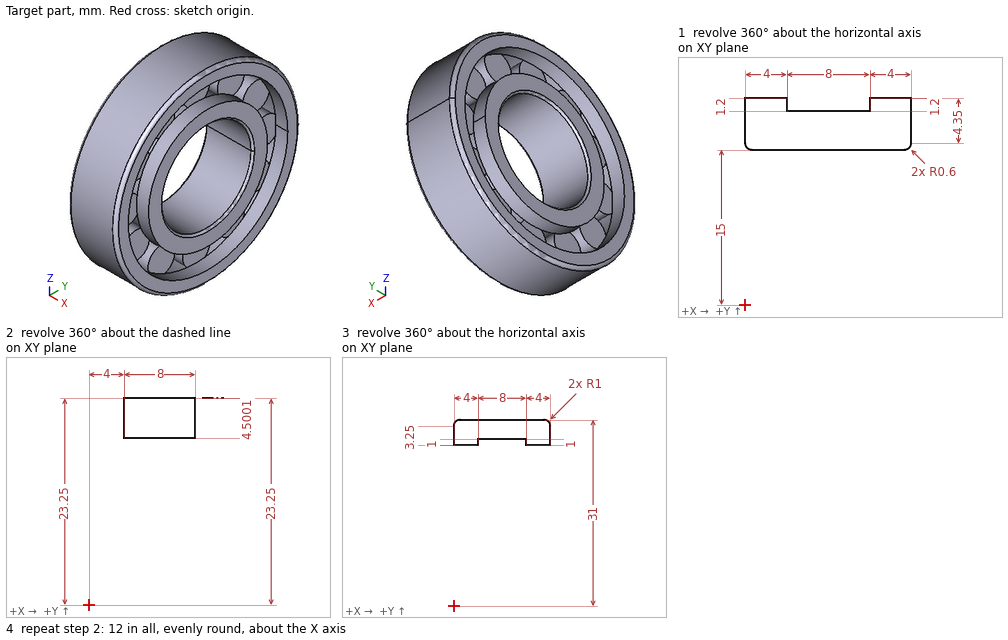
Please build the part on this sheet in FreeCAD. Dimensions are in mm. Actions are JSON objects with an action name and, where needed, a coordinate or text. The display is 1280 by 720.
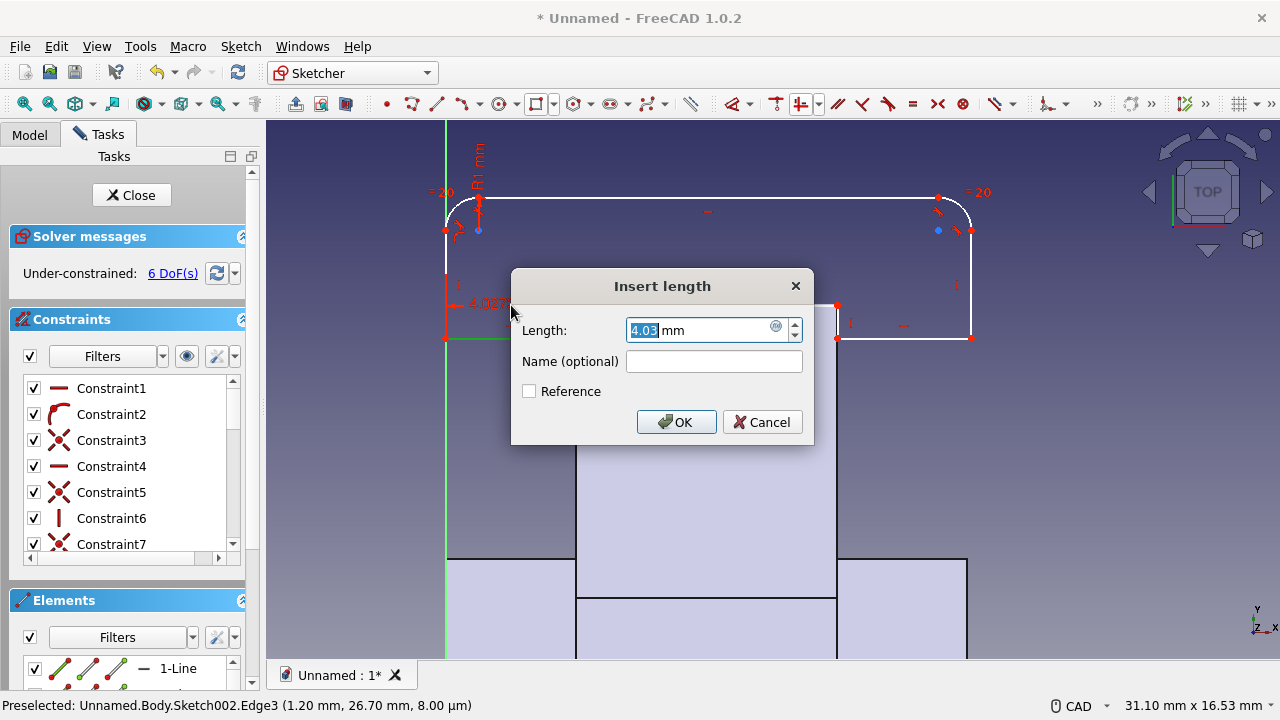
{"action": "type", "text": "4"}
{"action": "key", "text": "Return"}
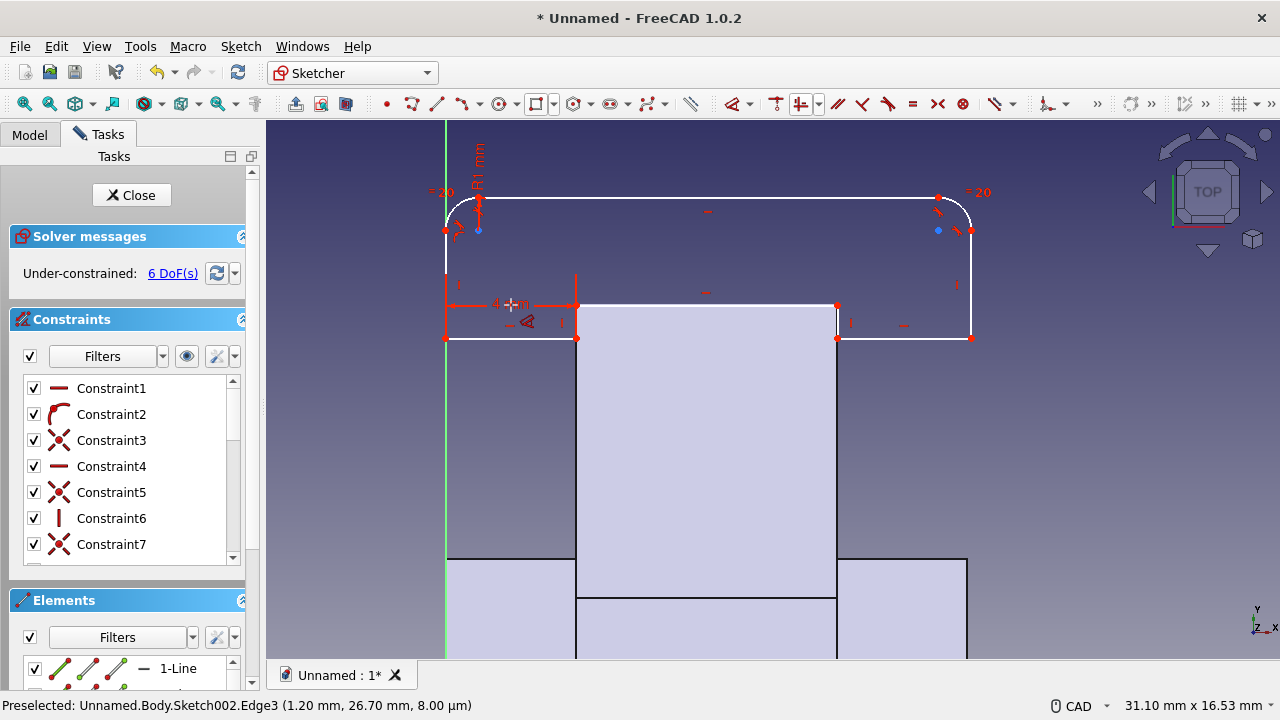
{"action": "scroll", "coordinate": [576, 329], "scroll_direction": "up", "scroll_amount": 2}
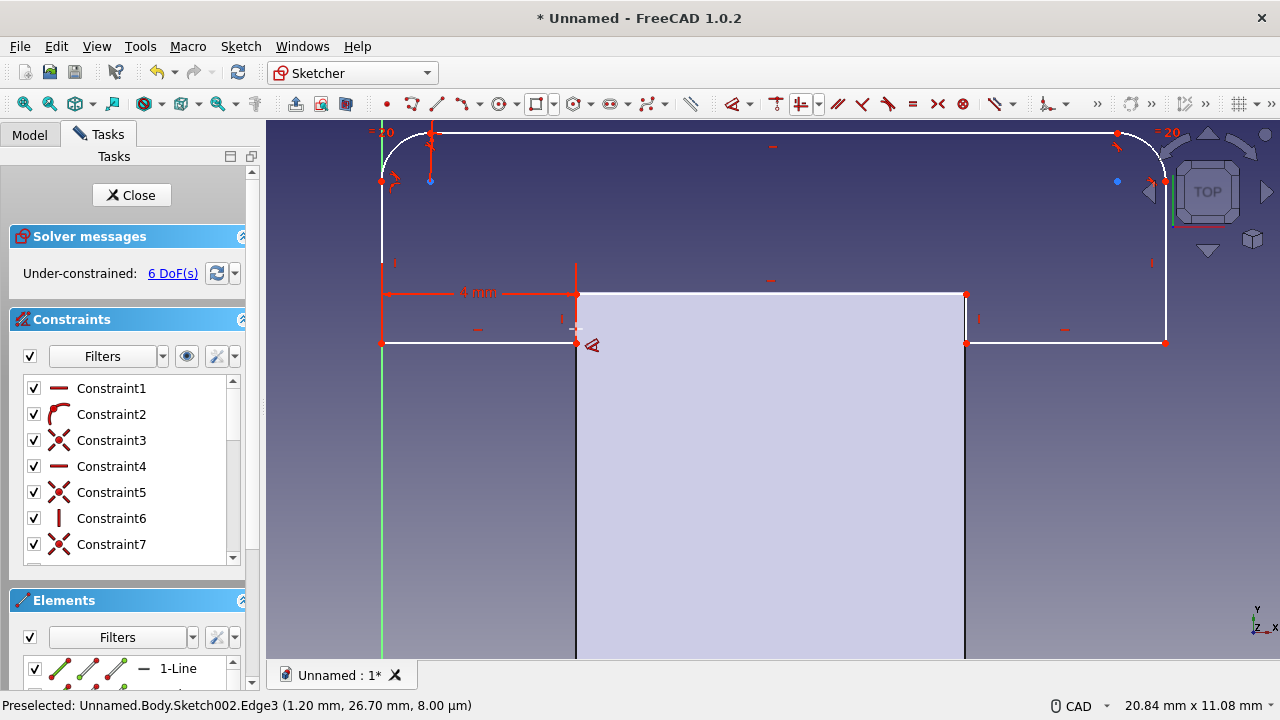
{"action": "left_click", "coordinate": [576, 328]}
{"action": "left_click", "coordinate": [542, 319]}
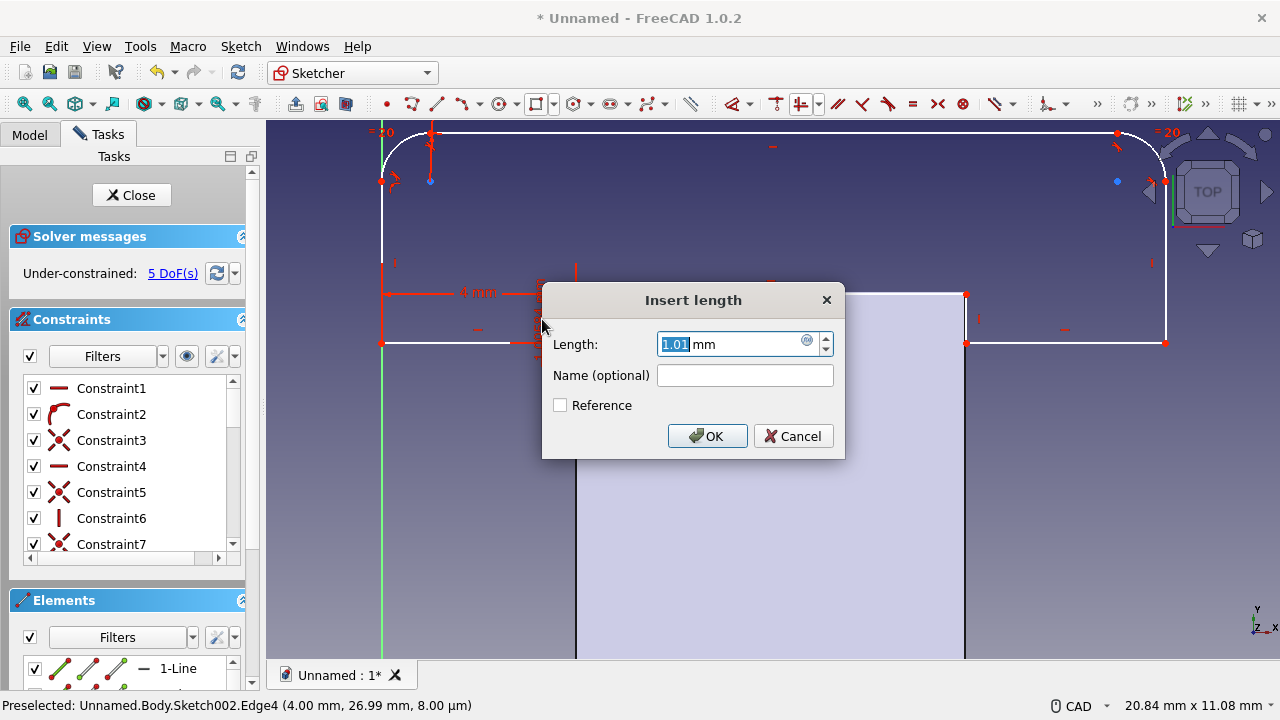
{"action": "type", "text": "1"}
{"action": "key", "text": "Return"}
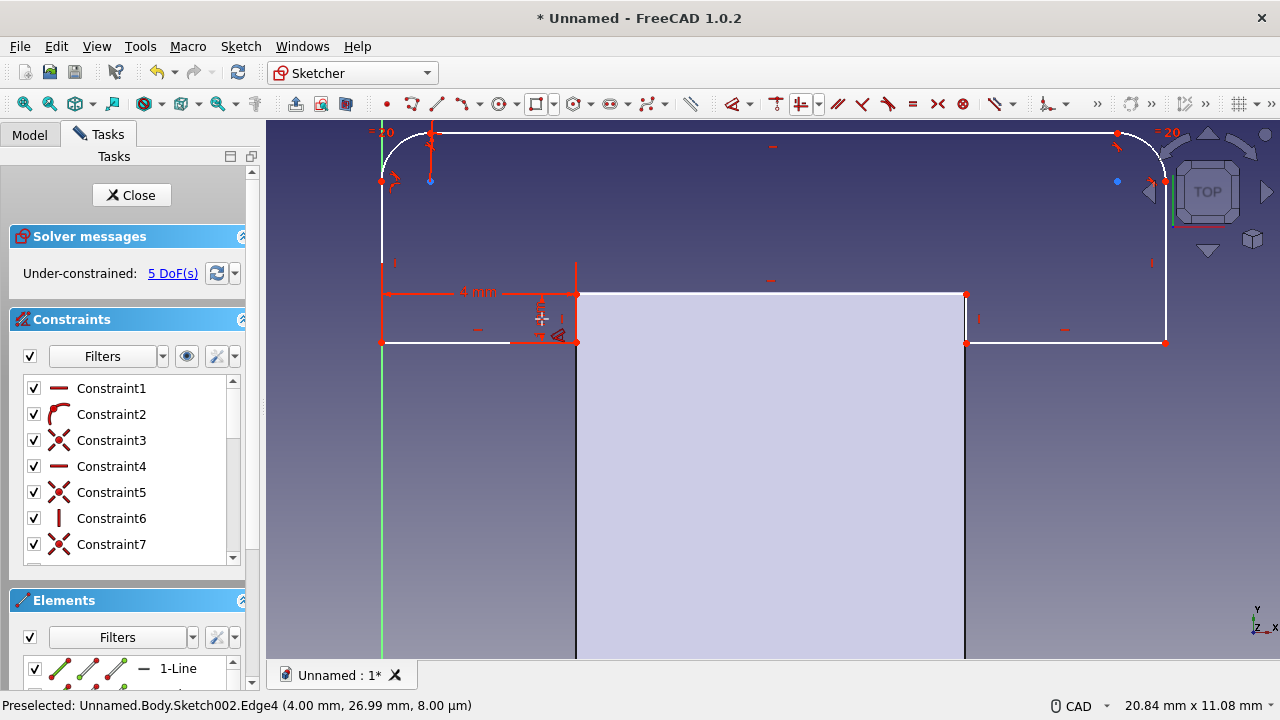
{"action": "scroll", "coordinate": [683, 226], "scroll_direction": "down", "scroll_amount": 7}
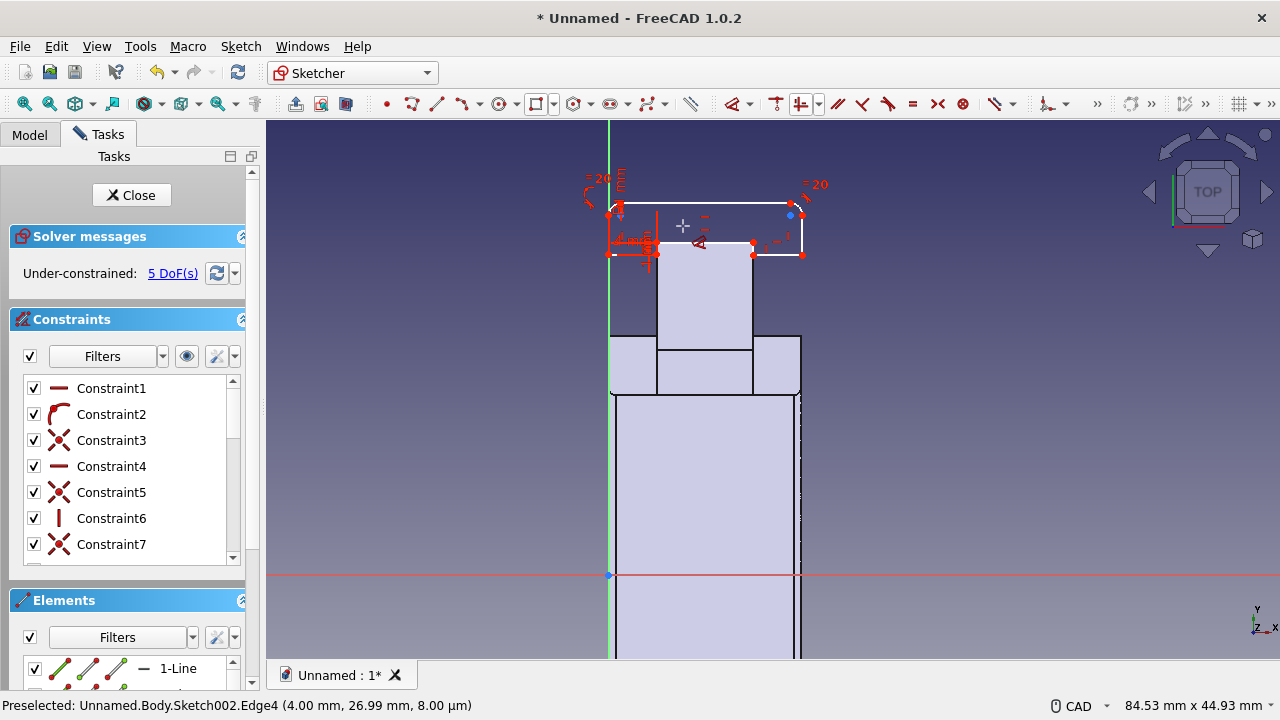
{"action": "left_click", "coordinate": [686, 243]}
{"action": "left_click", "coordinate": [705, 277]}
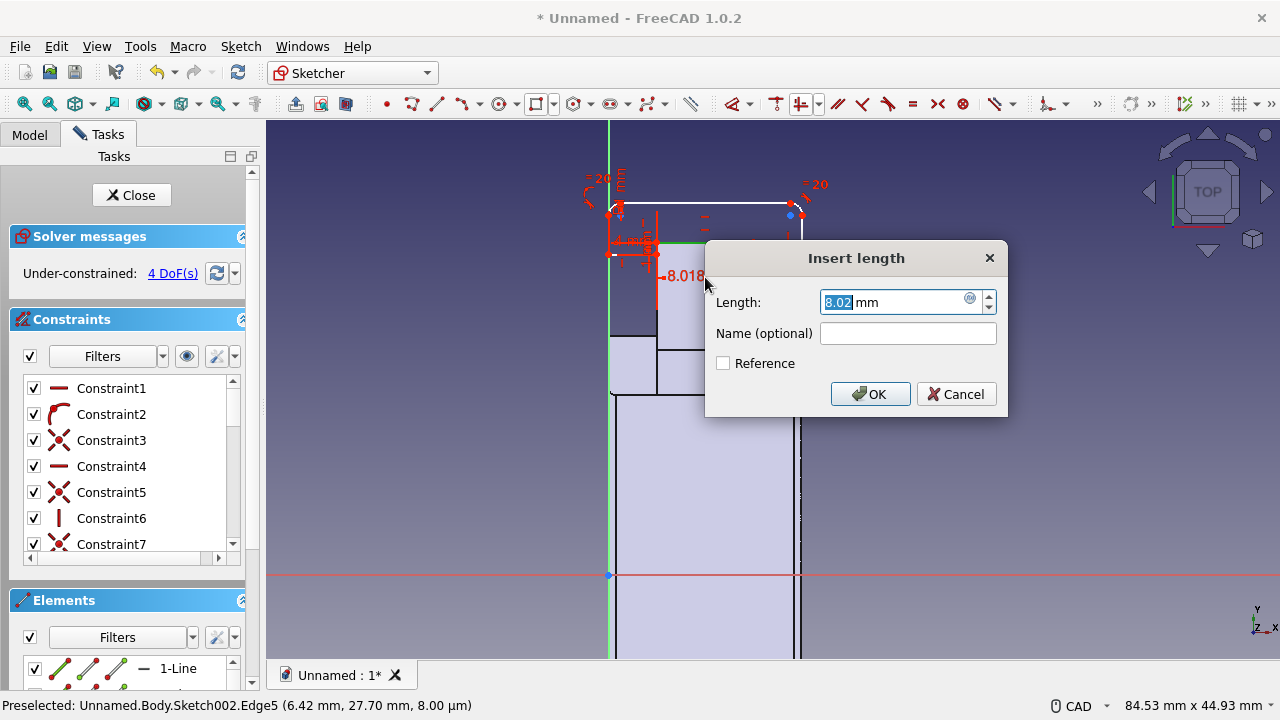
{"action": "type", "text": "8"}
{"action": "key", "text": "Return"}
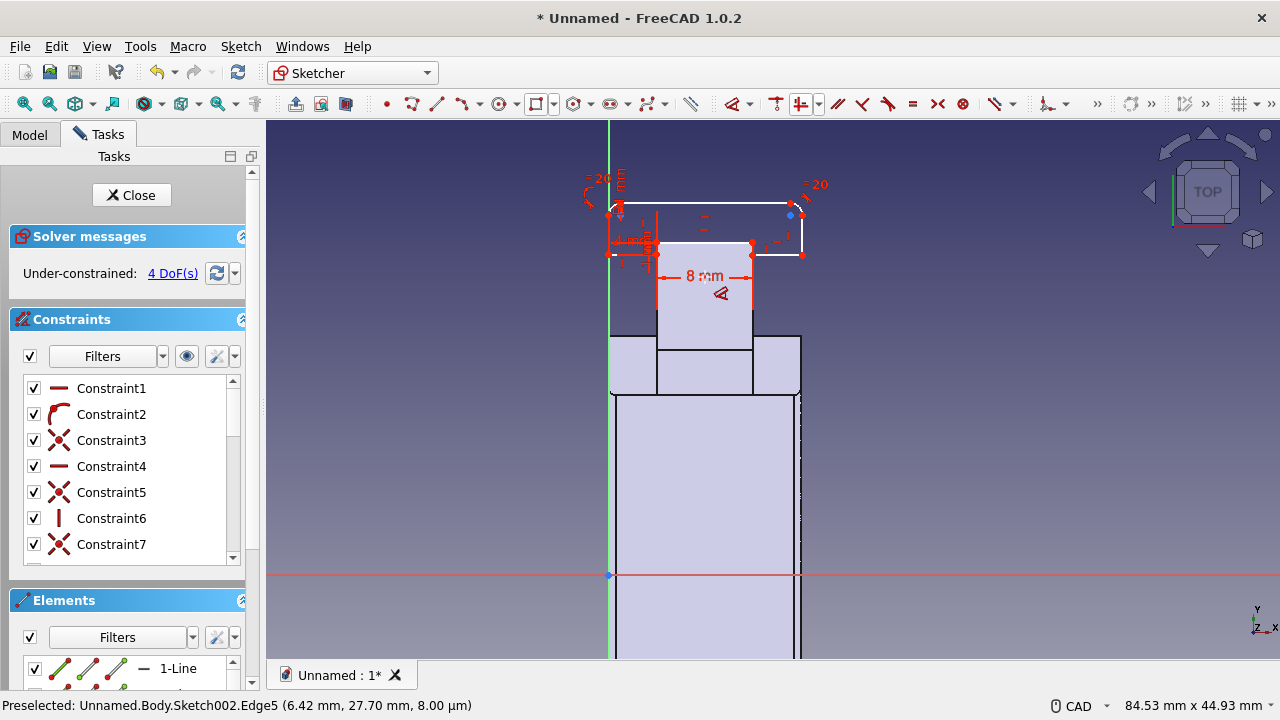
{"action": "scroll", "coordinate": [753, 249], "scroll_direction": "up", "scroll_amount": 6}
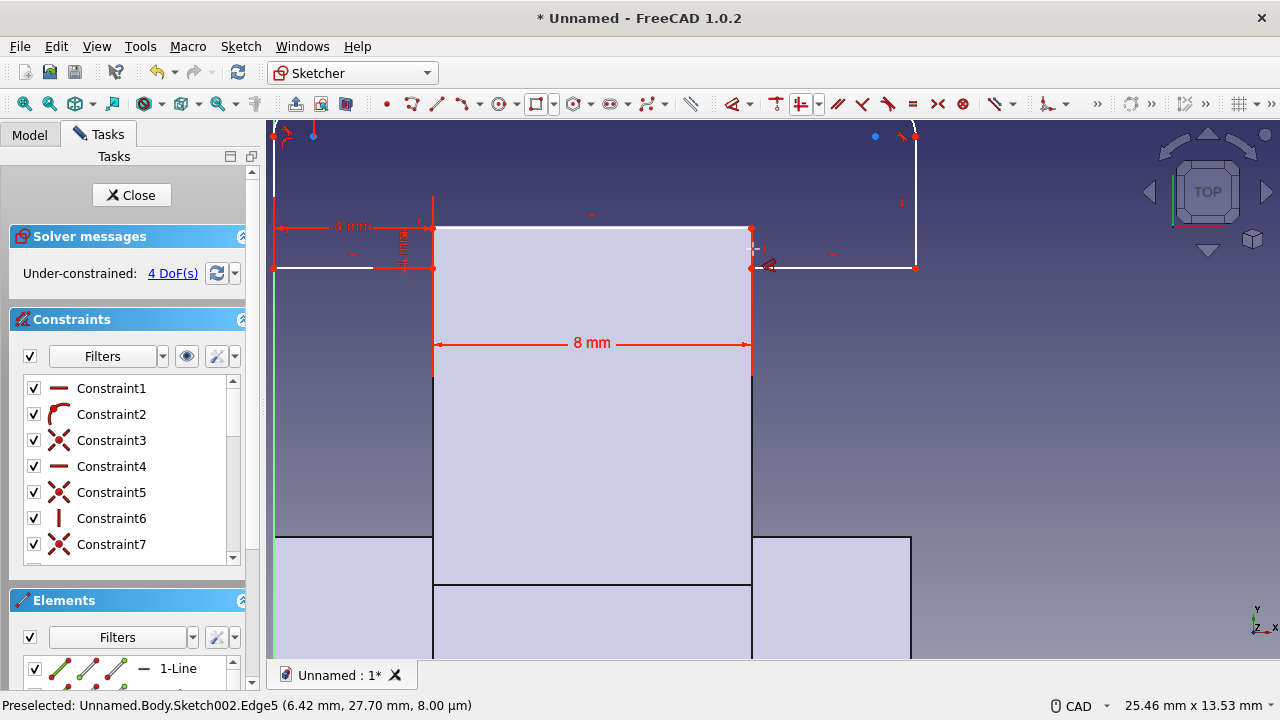
{"action": "left_click", "coordinate": [752, 248]}
{"action": "left_click", "coordinate": [786, 248]}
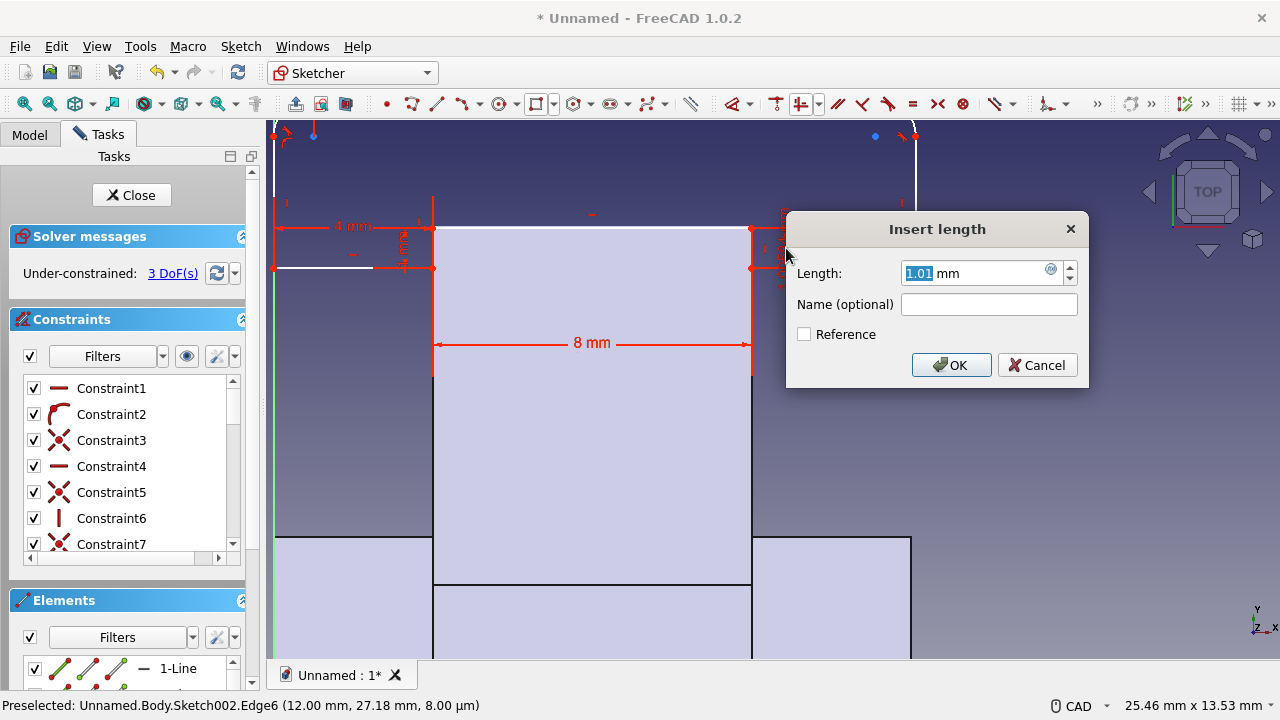
{"action": "type", "text": "1"}
{"action": "key", "text": "Return"}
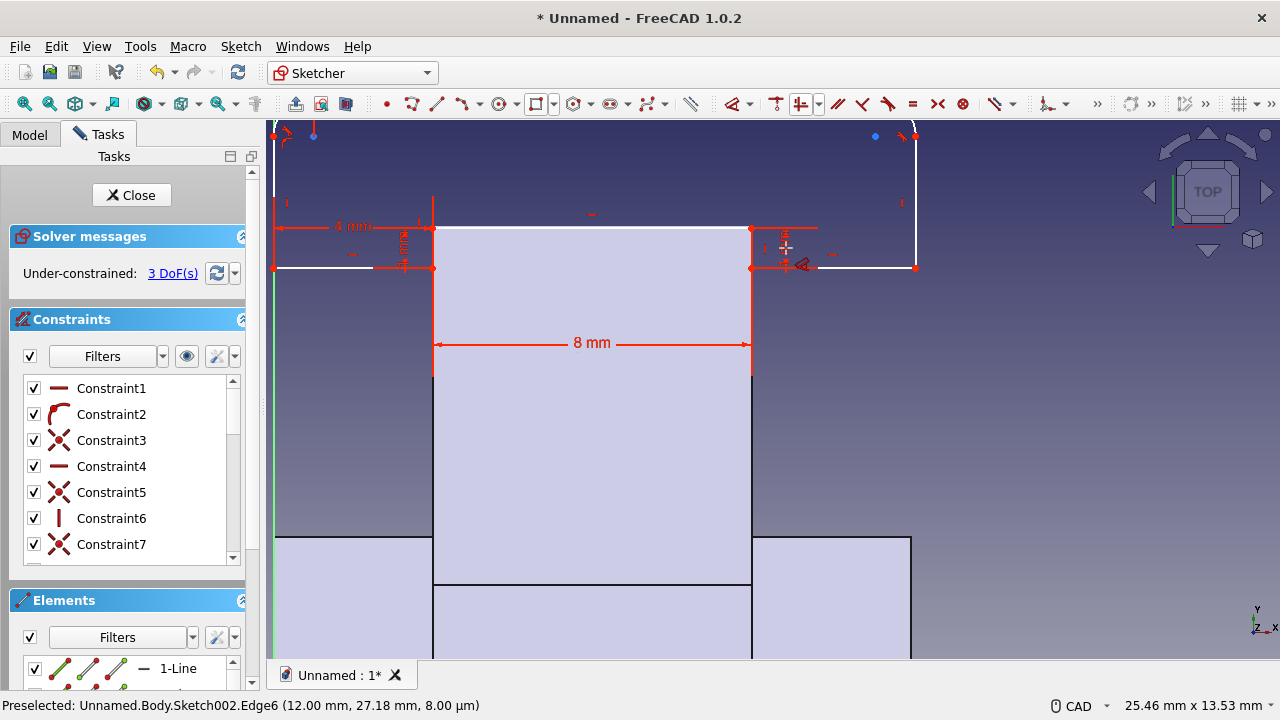
{"action": "left_click", "coordinate": [801, 268]}
{"action": "left_click", "coordinate": [871, 234]}